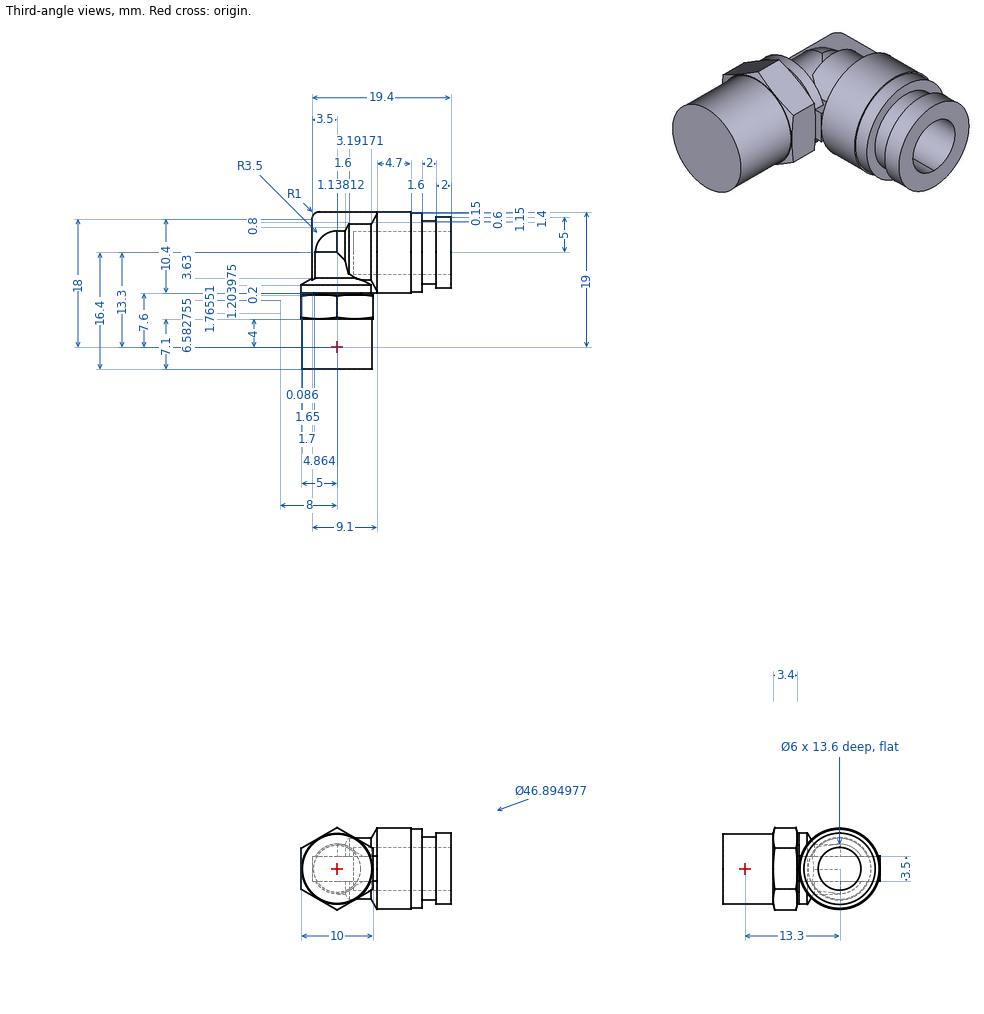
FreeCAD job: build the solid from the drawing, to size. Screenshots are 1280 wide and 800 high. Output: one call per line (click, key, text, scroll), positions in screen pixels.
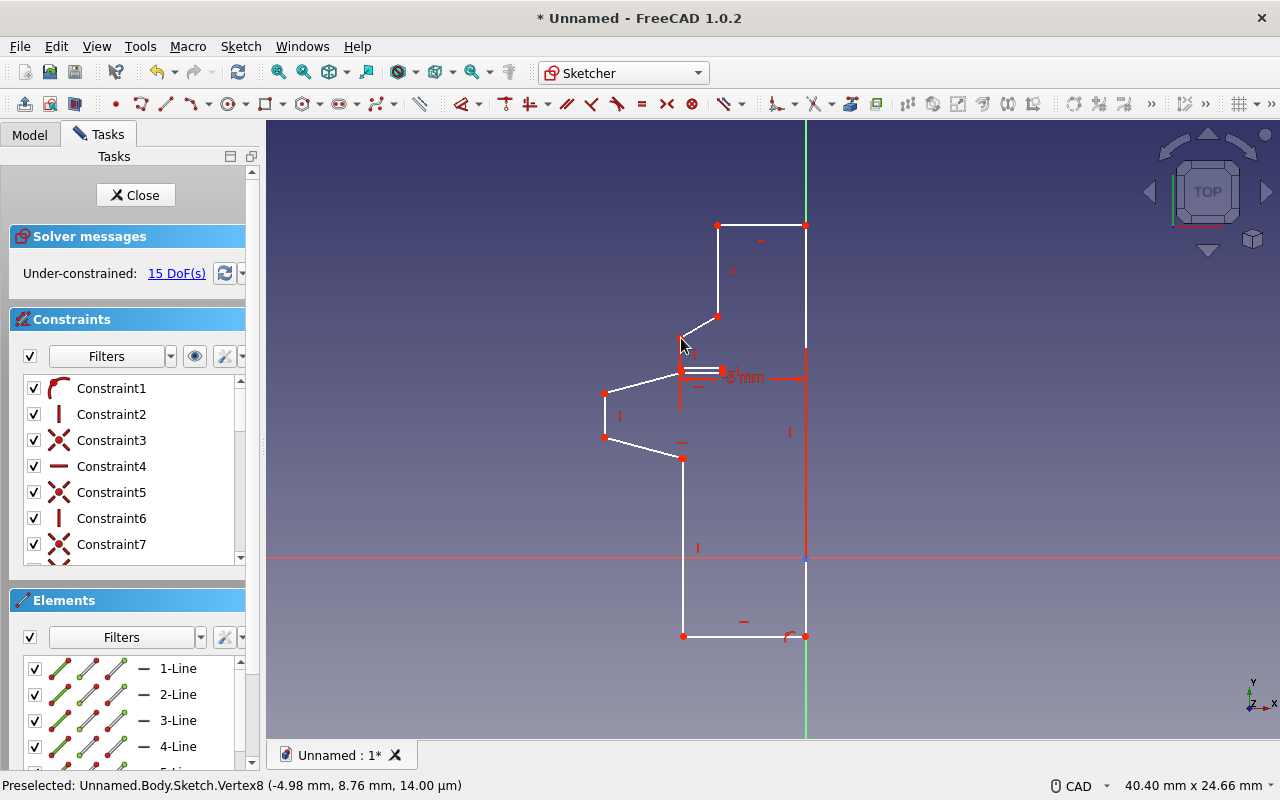
click(605, 393)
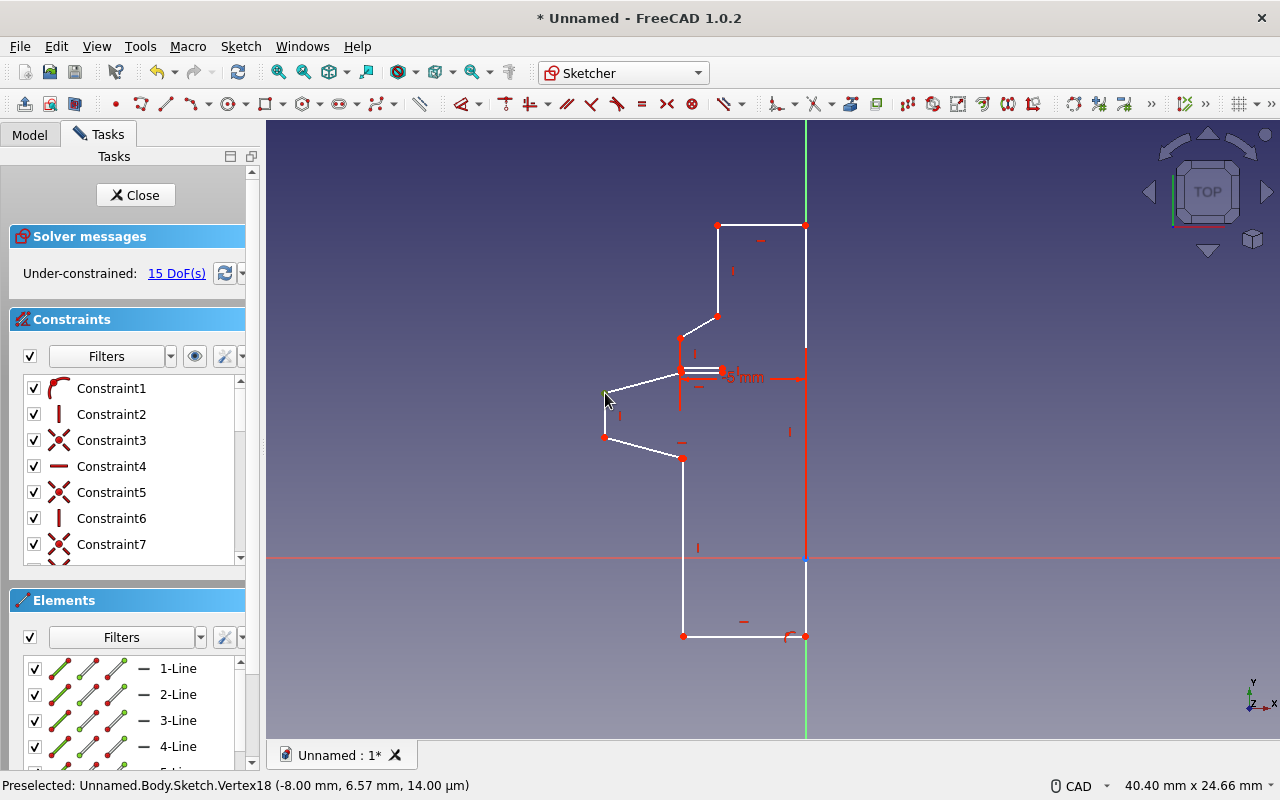
key(l)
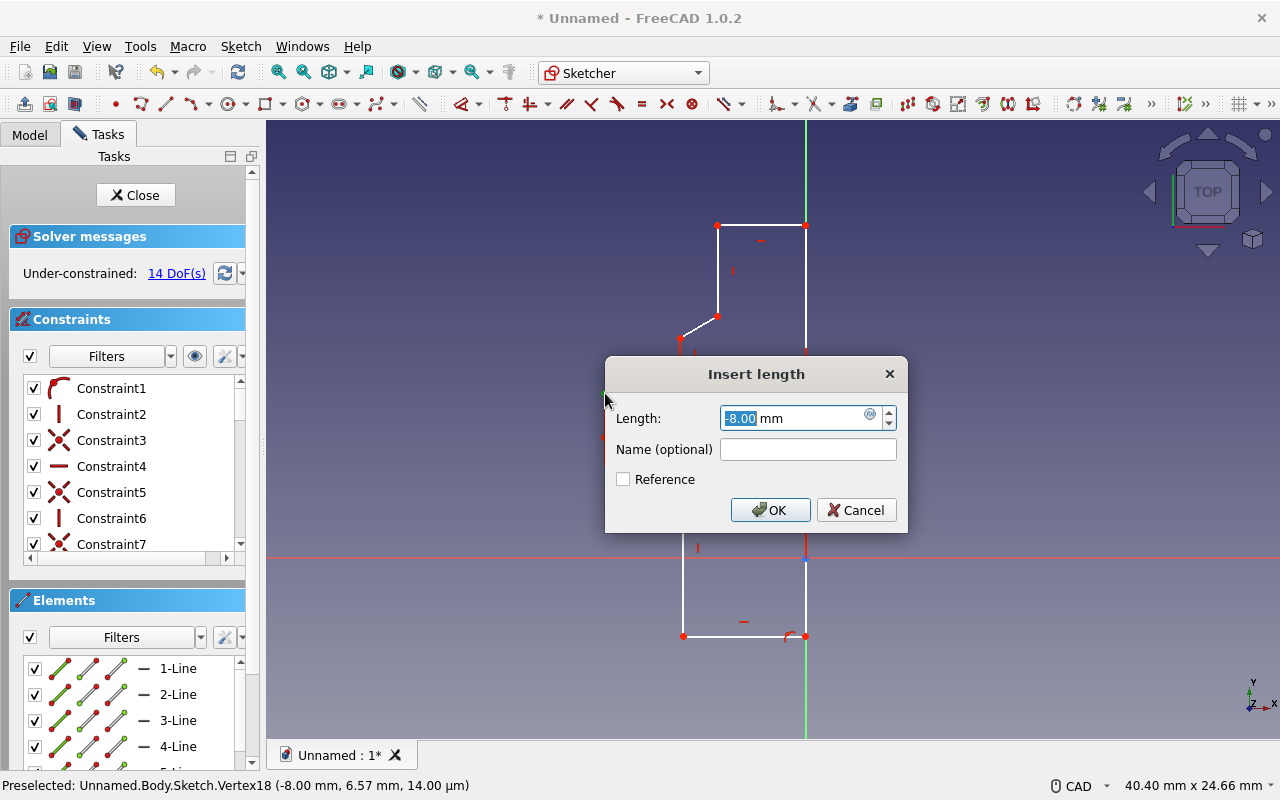
text(-8)
key(Return)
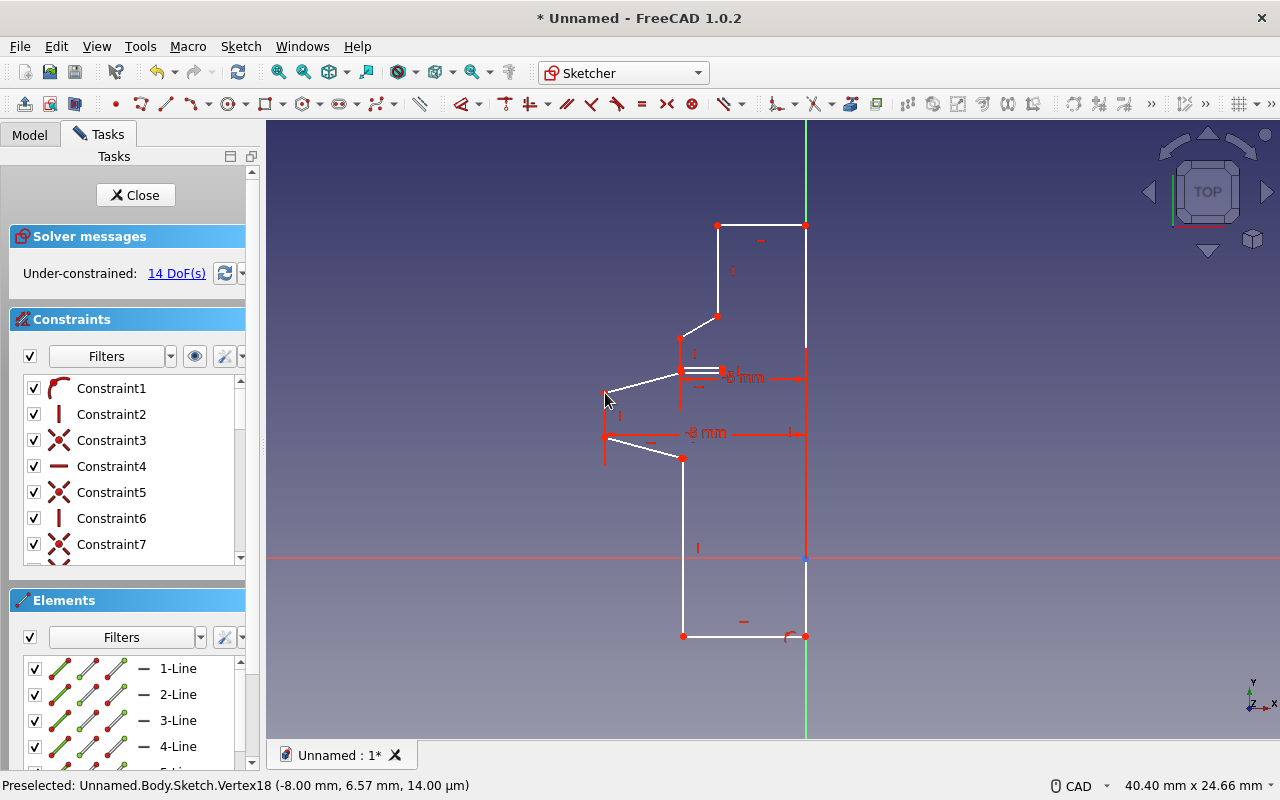
scroll(681, 458, up, 9)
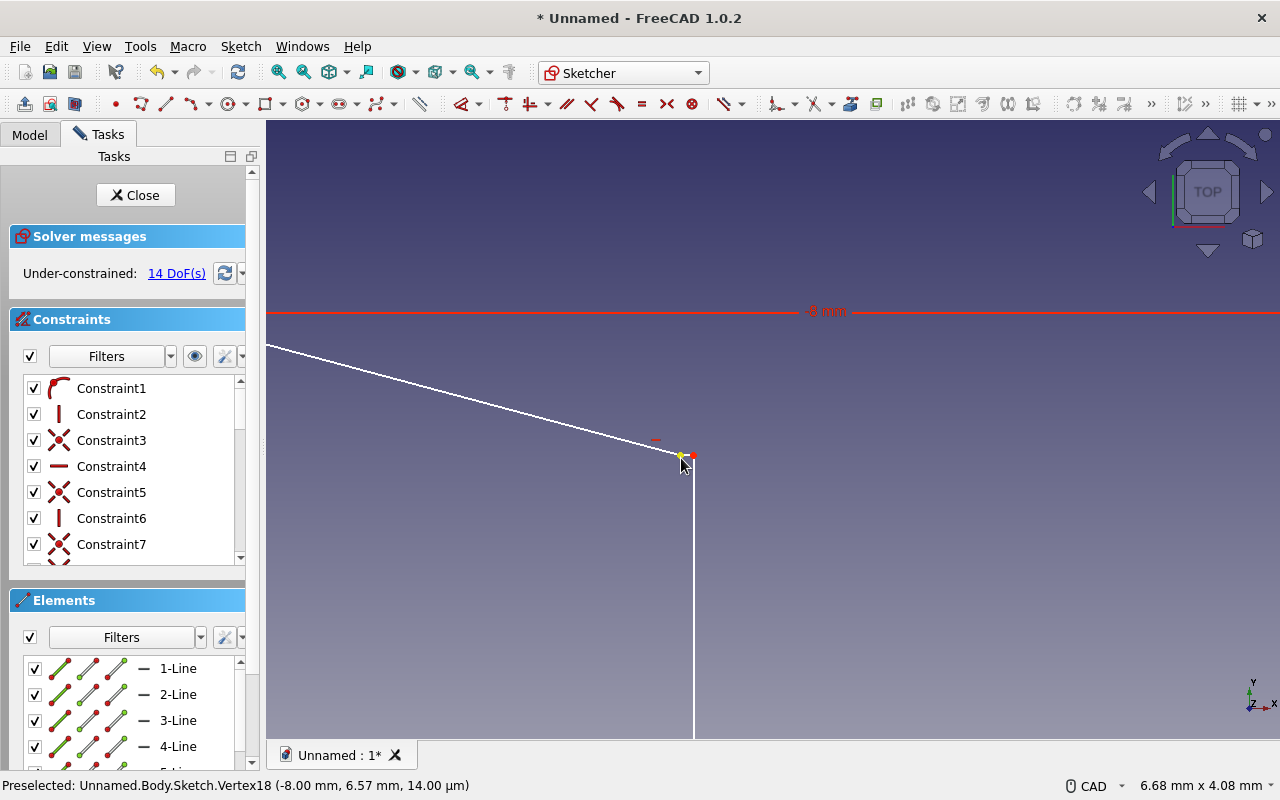
click(681, 455)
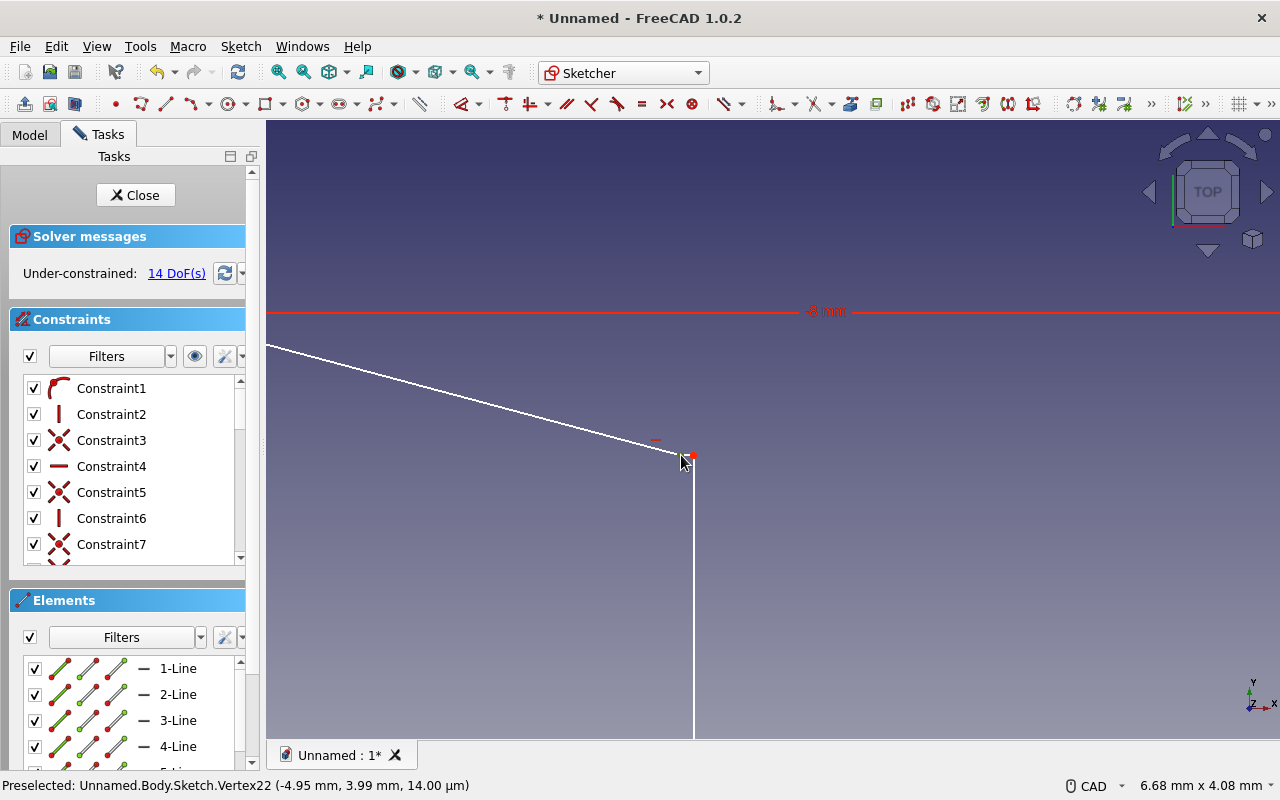
key(i)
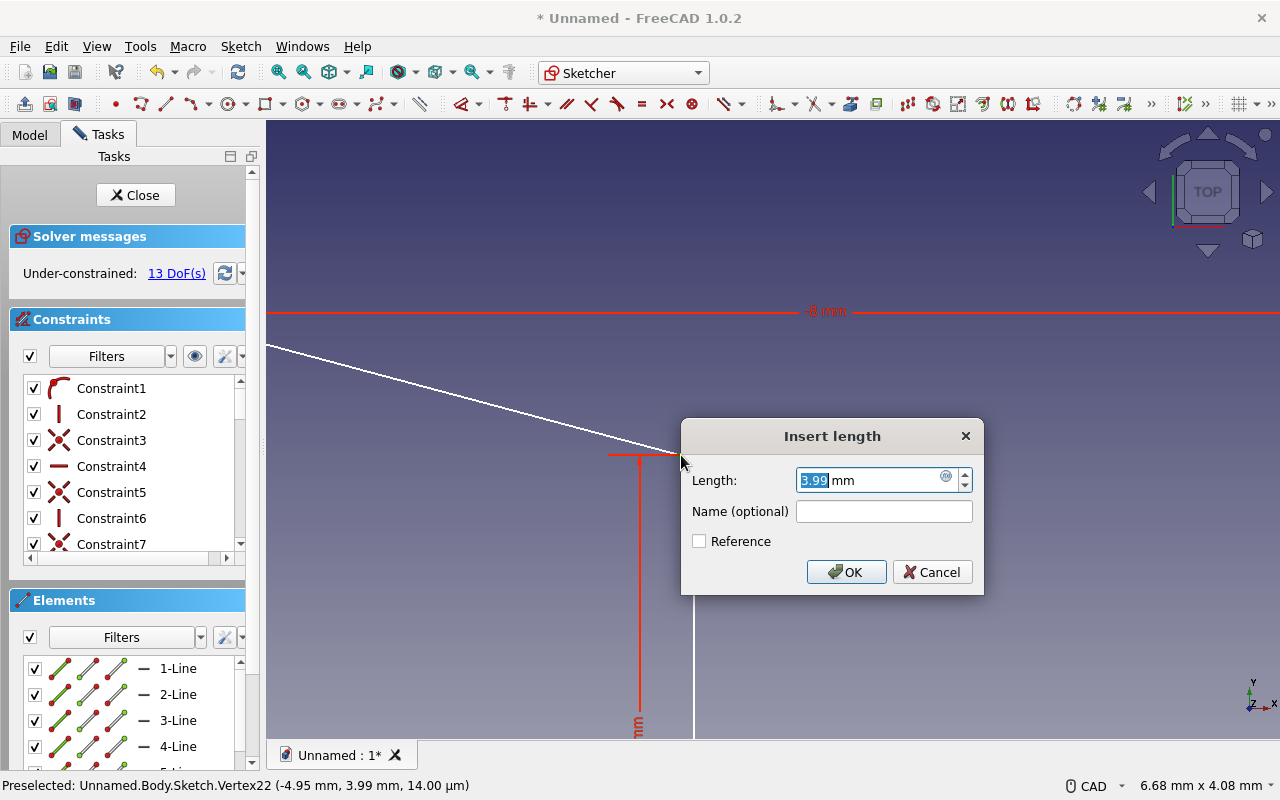
text(4)
key(Return)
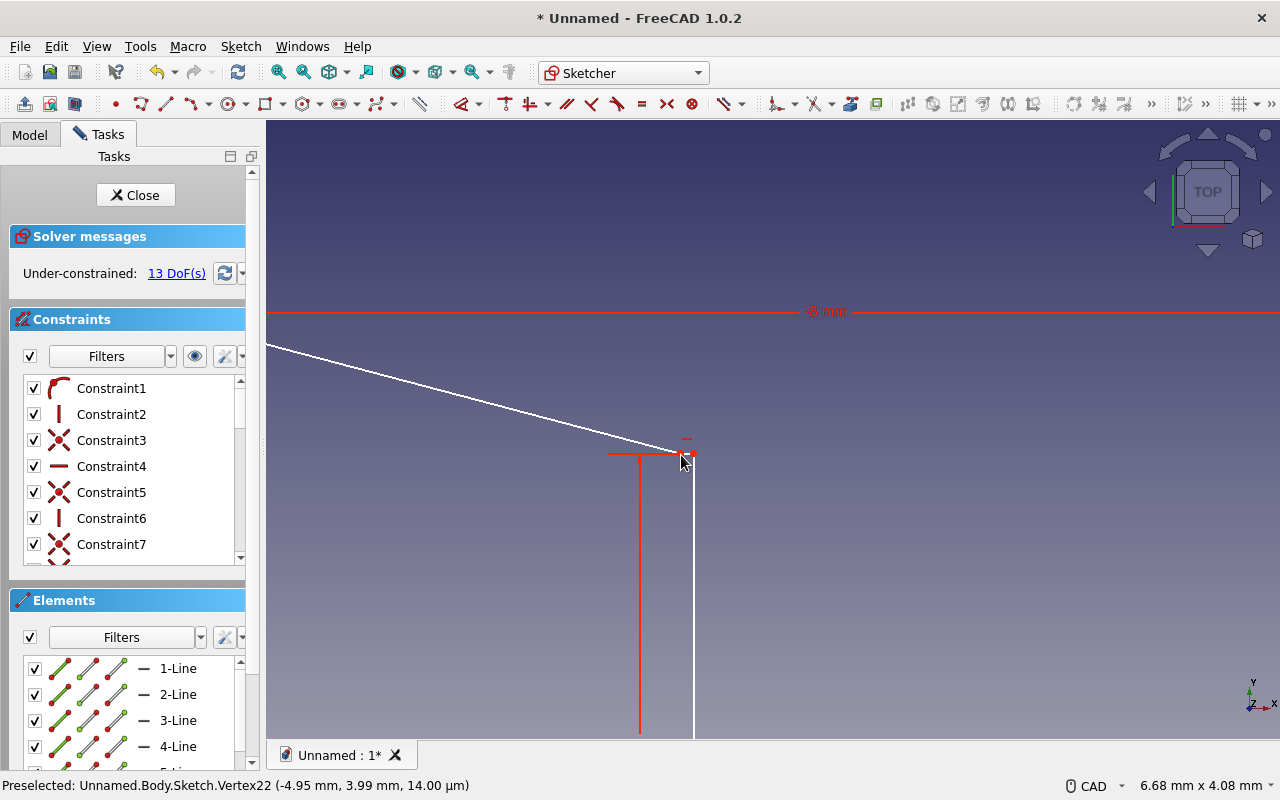
scroll(681, 458, down, 9)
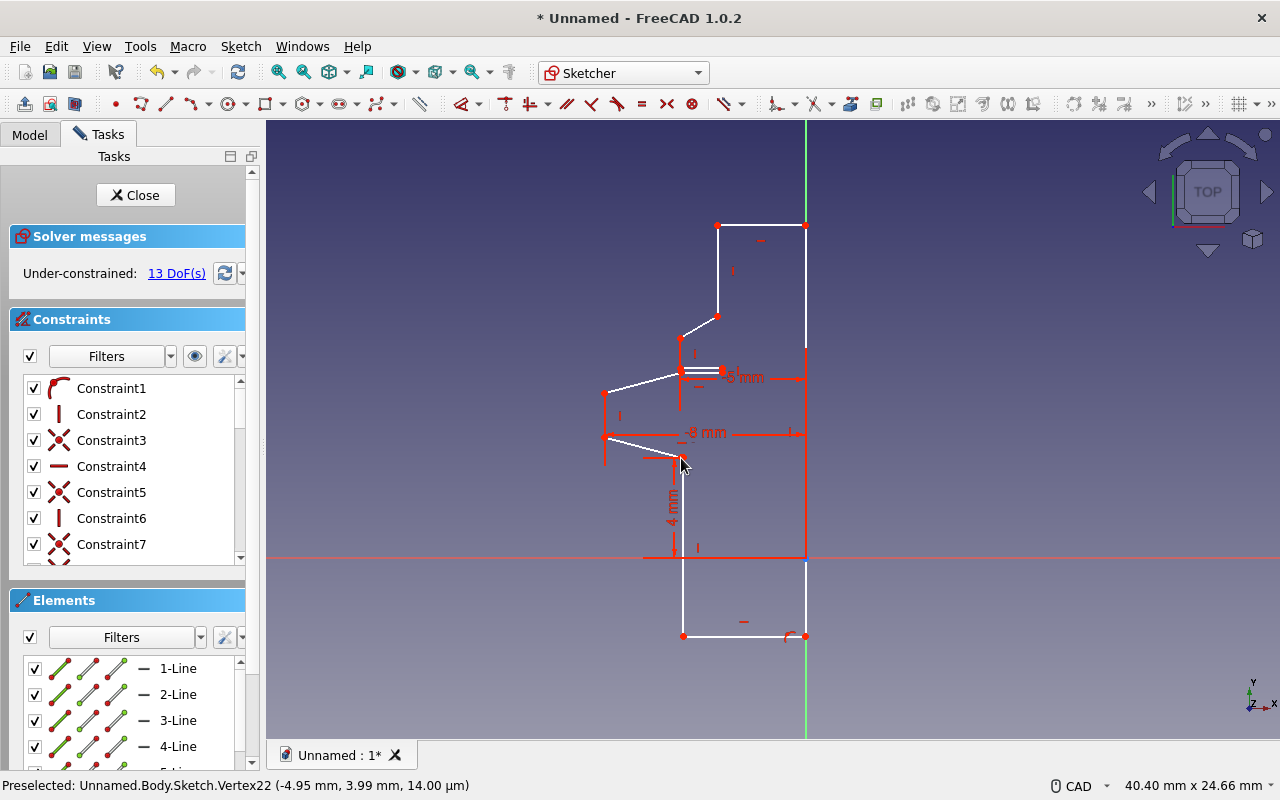
click(779, 225)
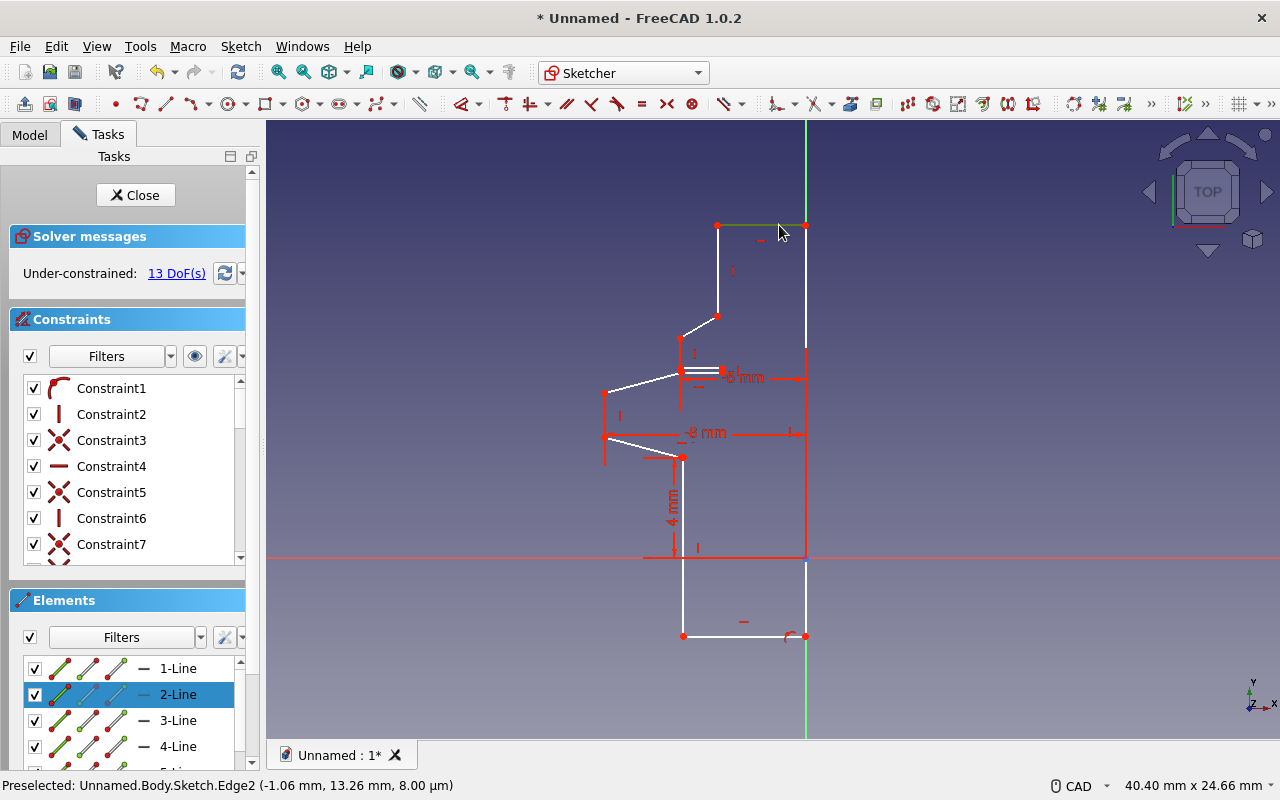
key(l)